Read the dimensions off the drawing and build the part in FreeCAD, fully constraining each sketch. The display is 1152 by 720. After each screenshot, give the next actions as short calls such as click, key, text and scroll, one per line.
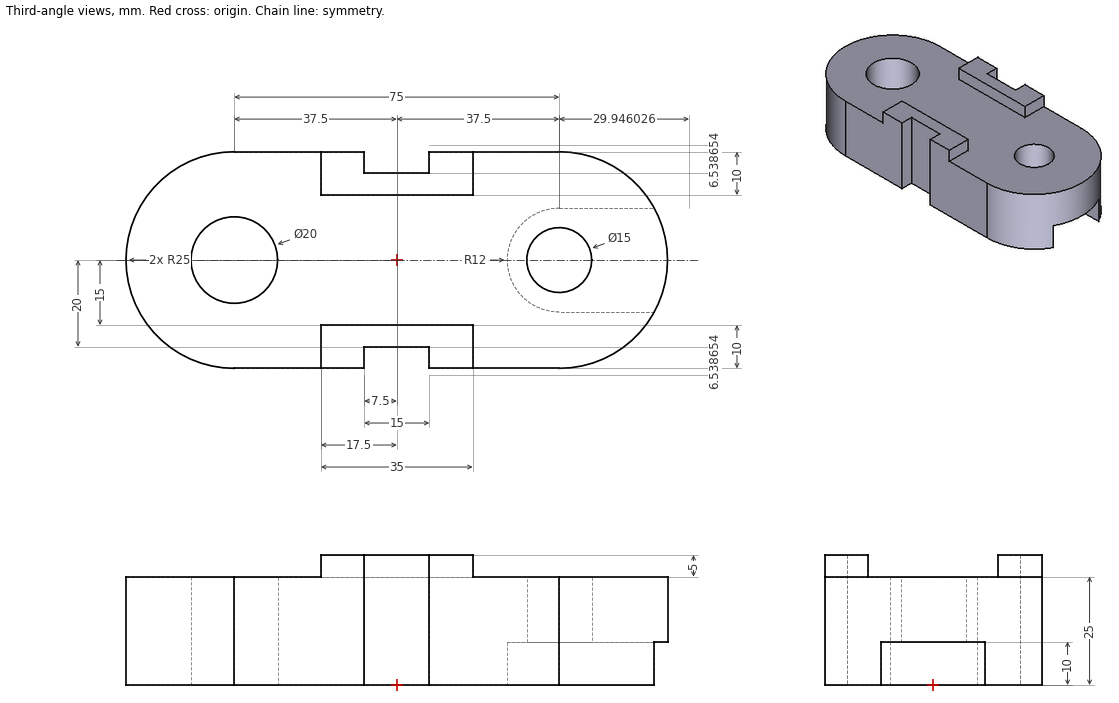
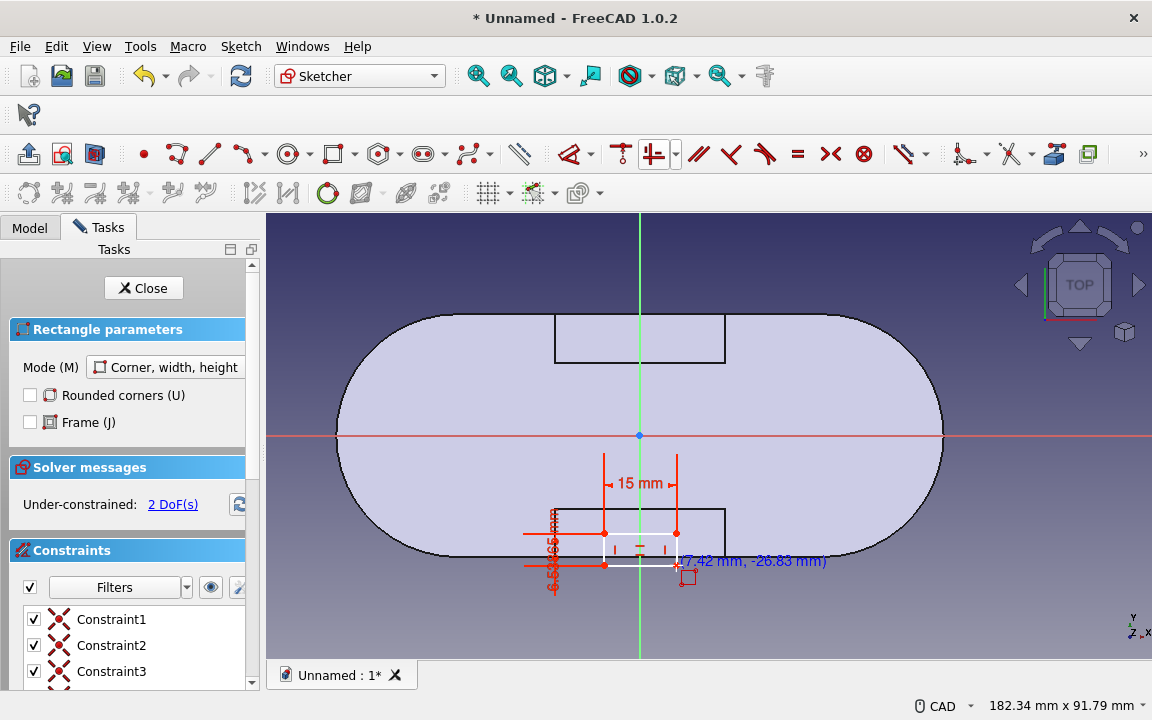
click(604, 307)
move(676, 338)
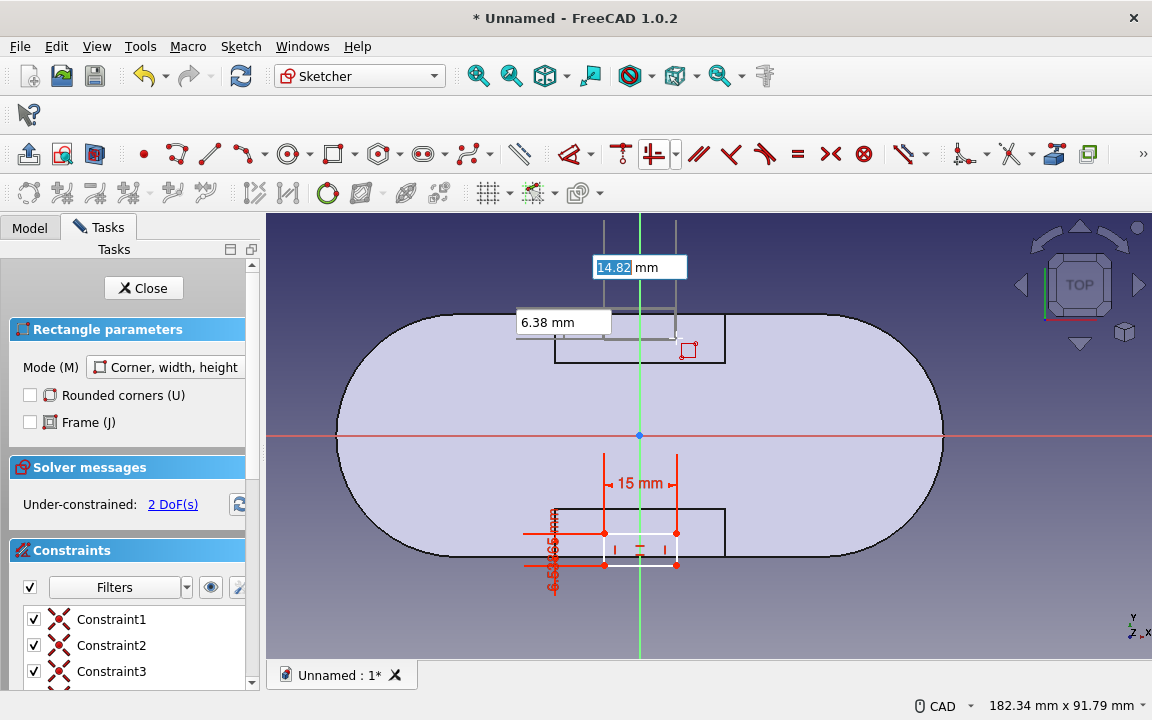
text(15)
key(Tab)
text(6.538654)
key(Return)
key(Escape)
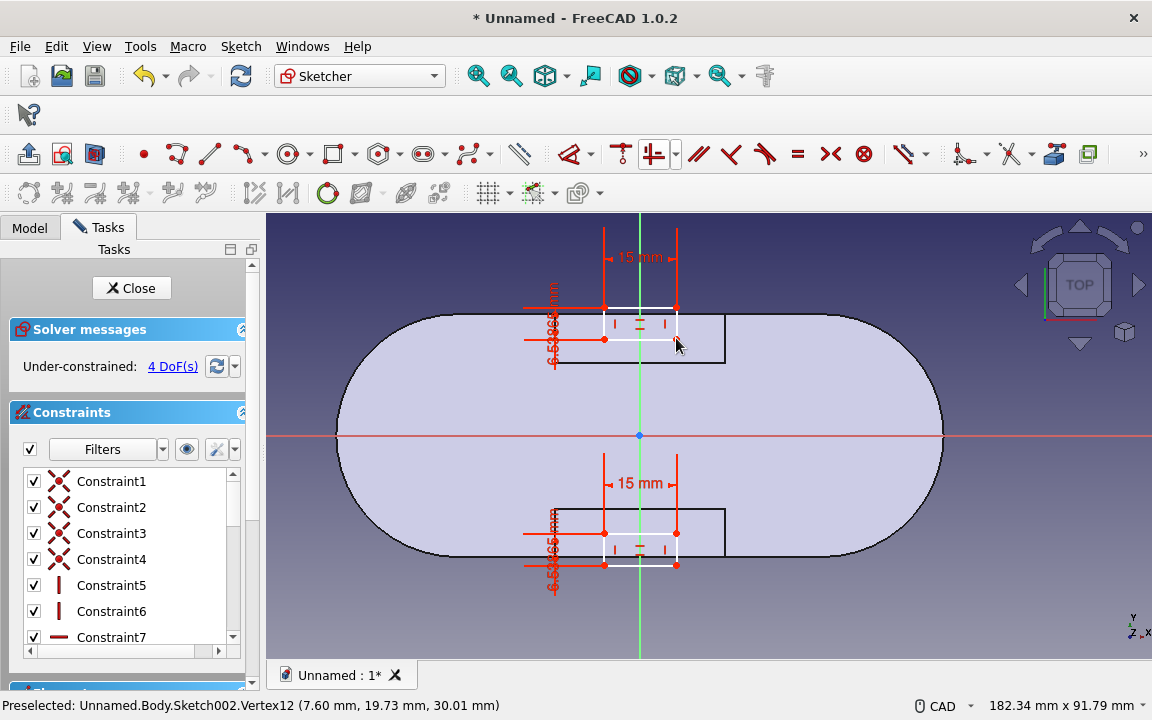
click(604, 566)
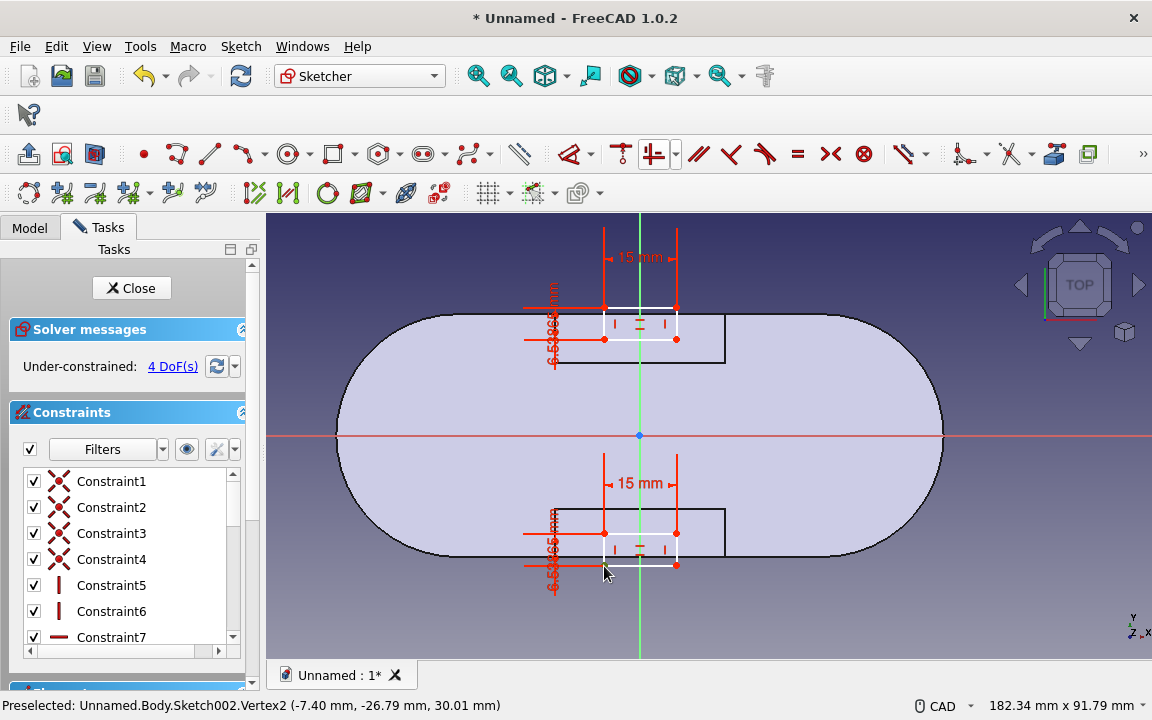
click(604, 308)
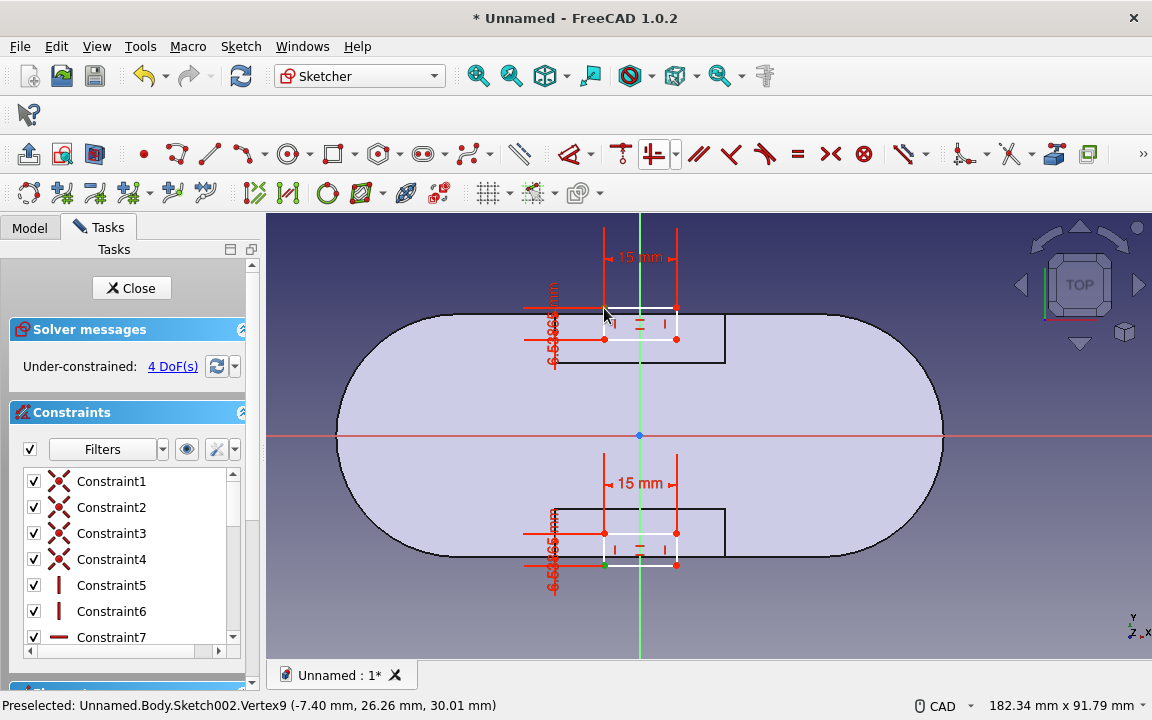
click(344, 436)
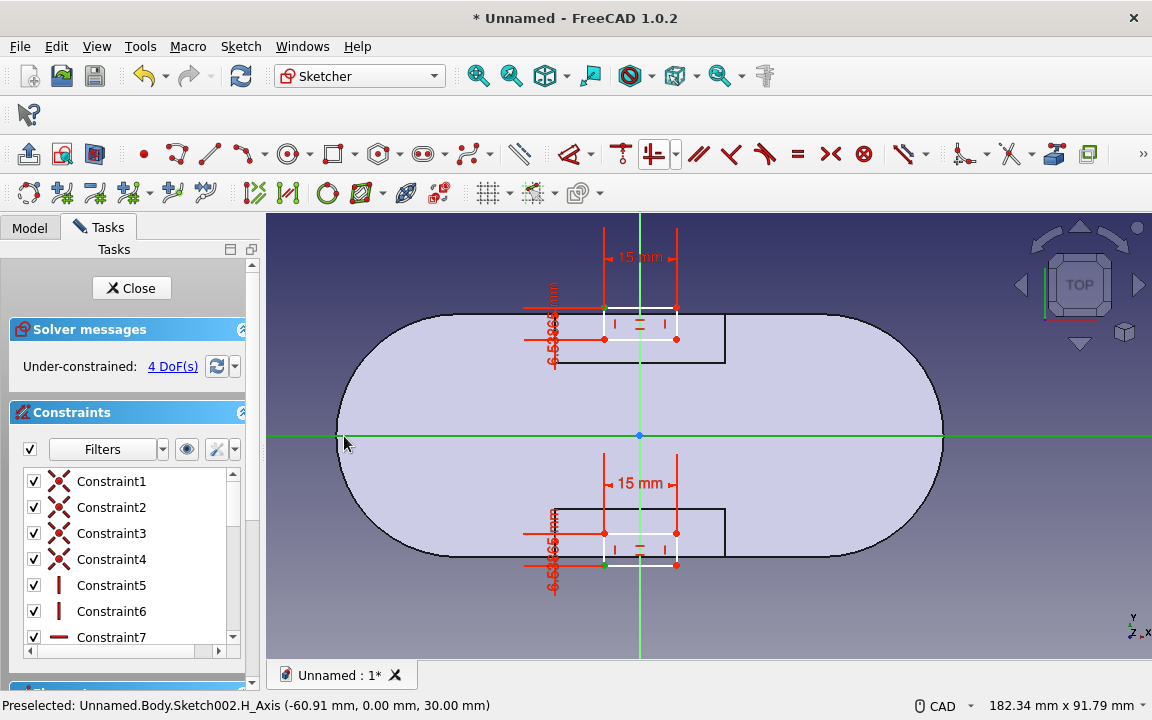
click(831, 154)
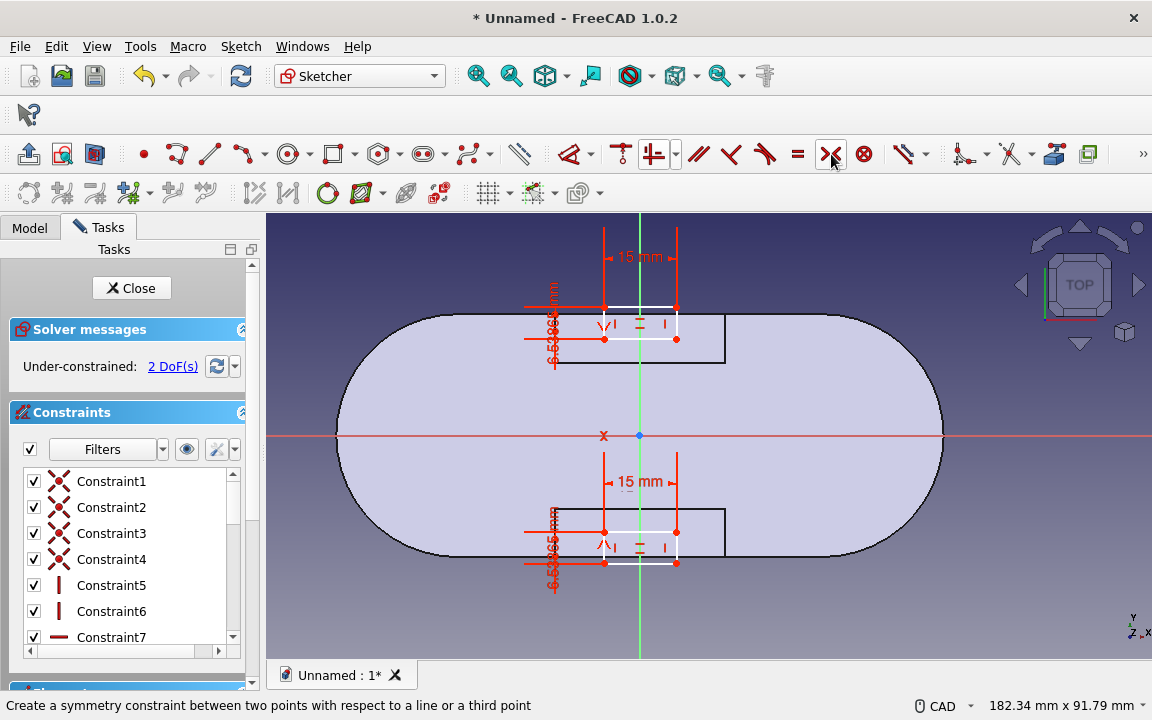
click(568, 154)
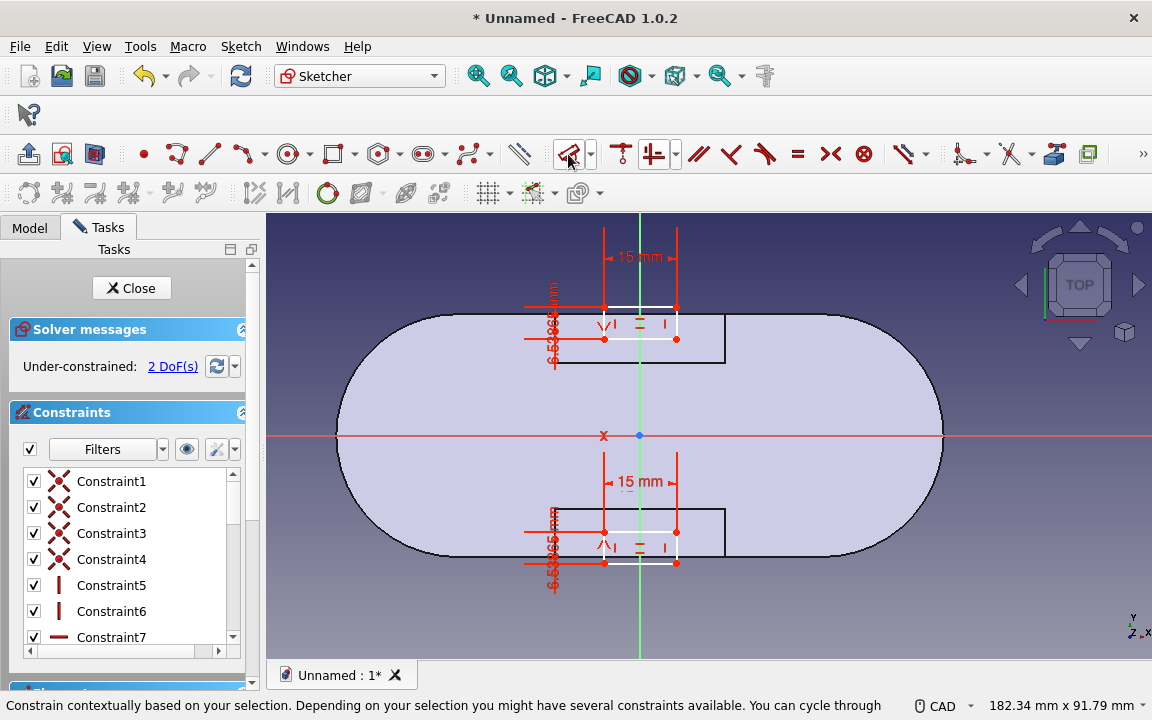
click(604, 532)
click(570, 484)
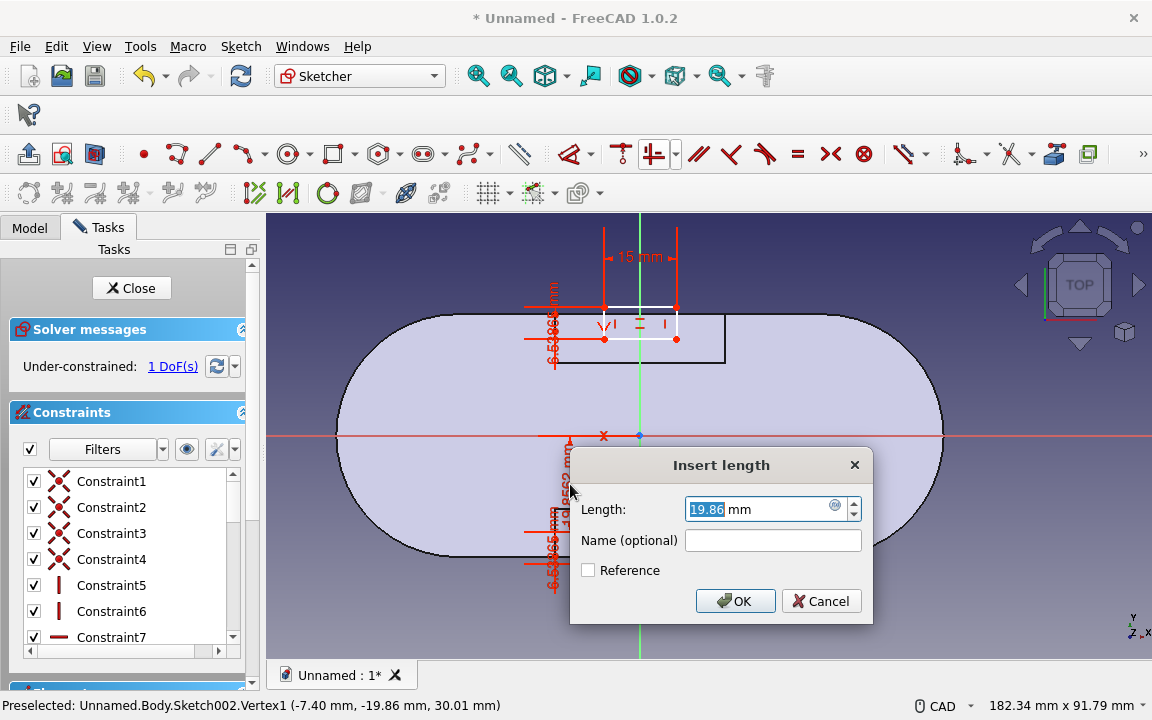
text(20)
key(Return)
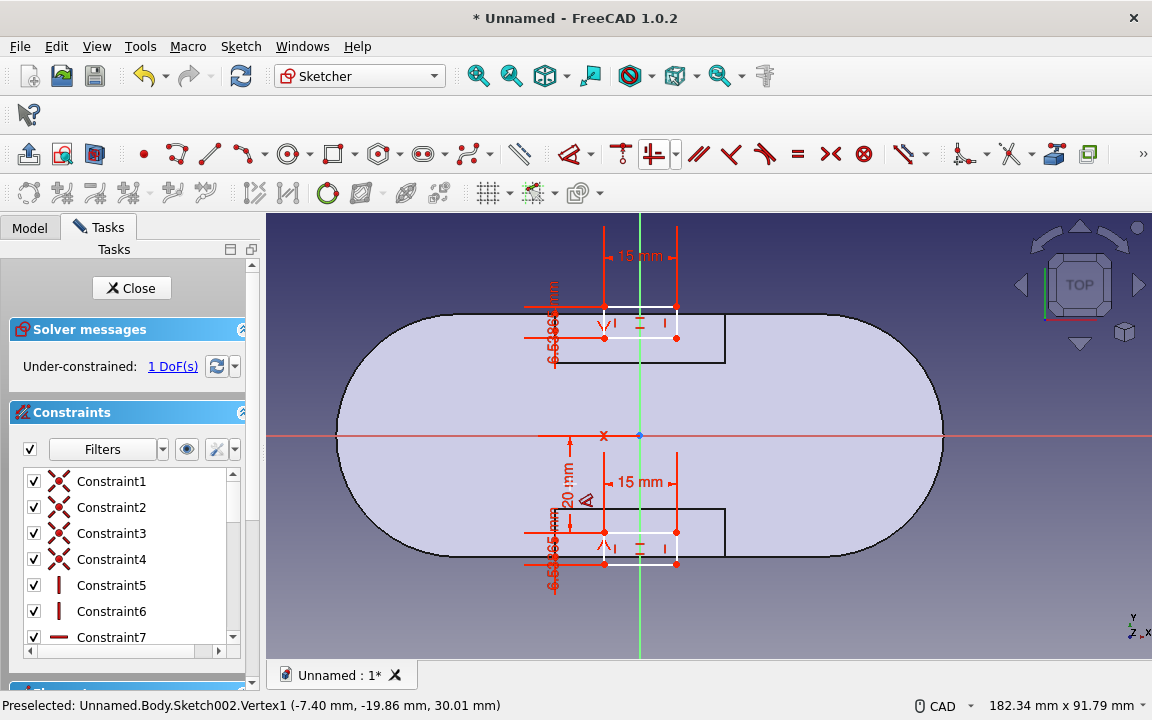
click(604, 533)
click(622, 402)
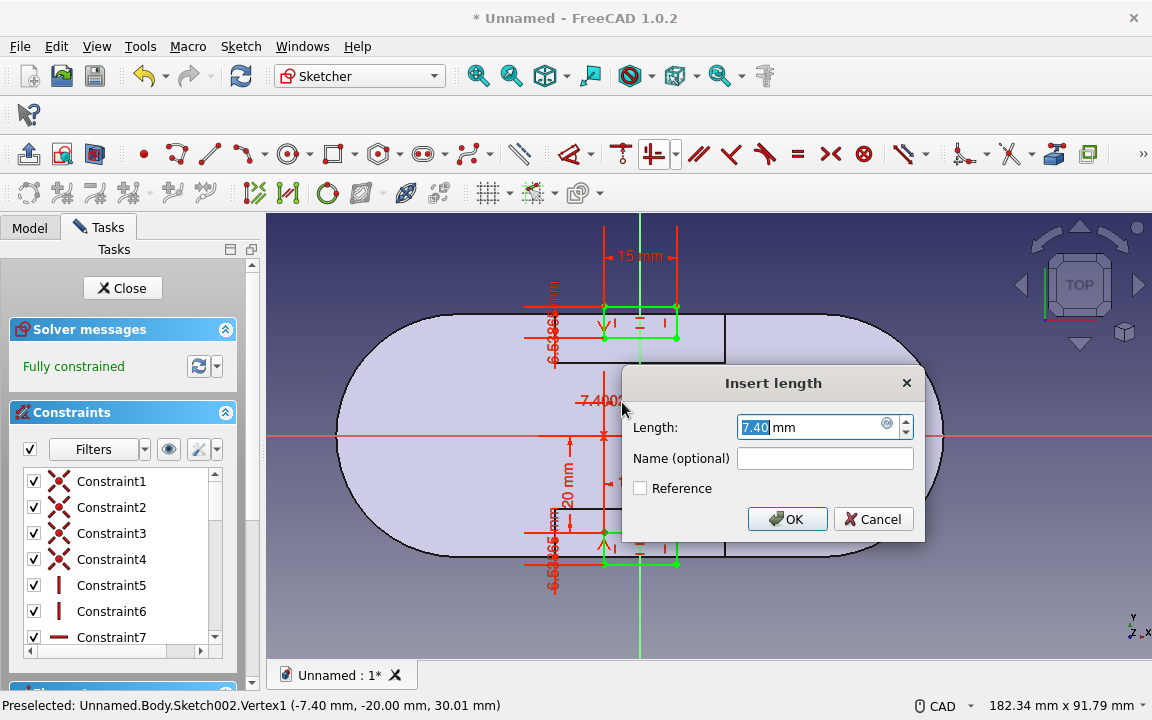
text(7.5)
key(Return)
key(Escape)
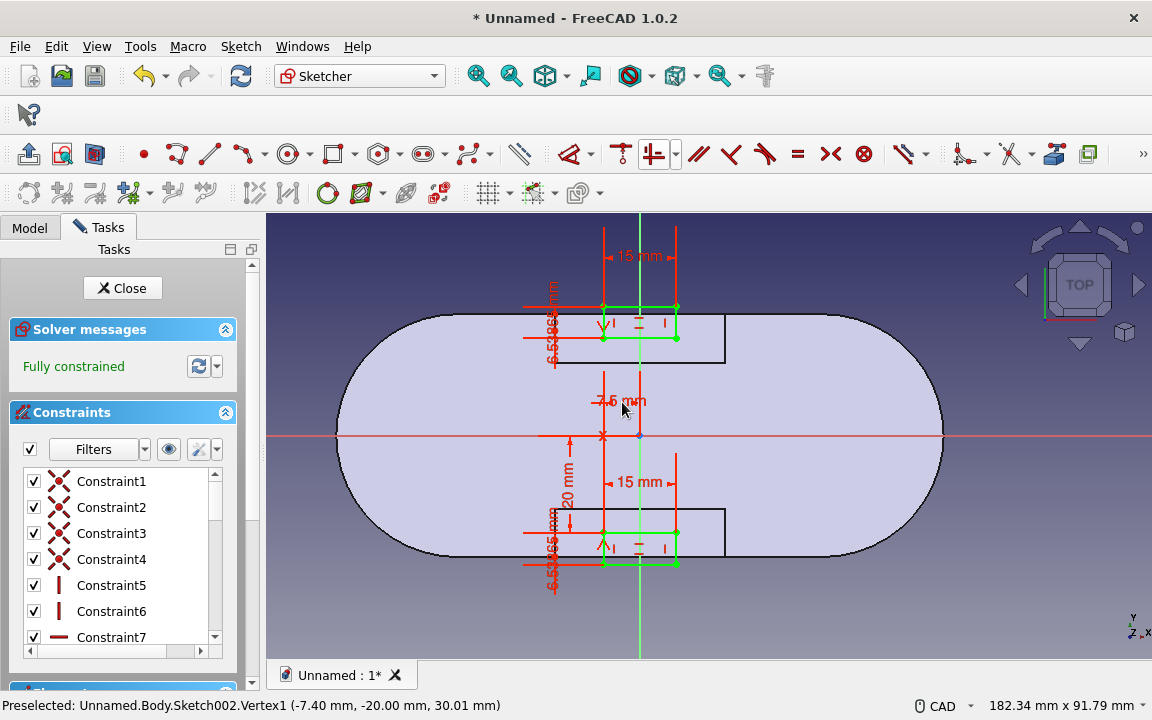
click(123, 288)